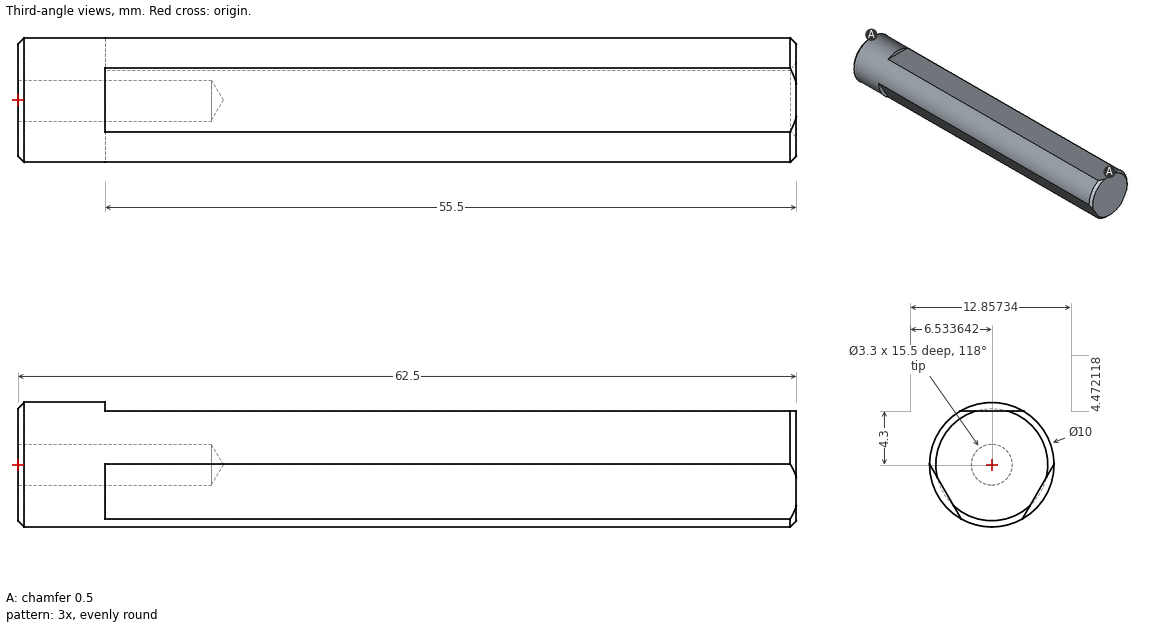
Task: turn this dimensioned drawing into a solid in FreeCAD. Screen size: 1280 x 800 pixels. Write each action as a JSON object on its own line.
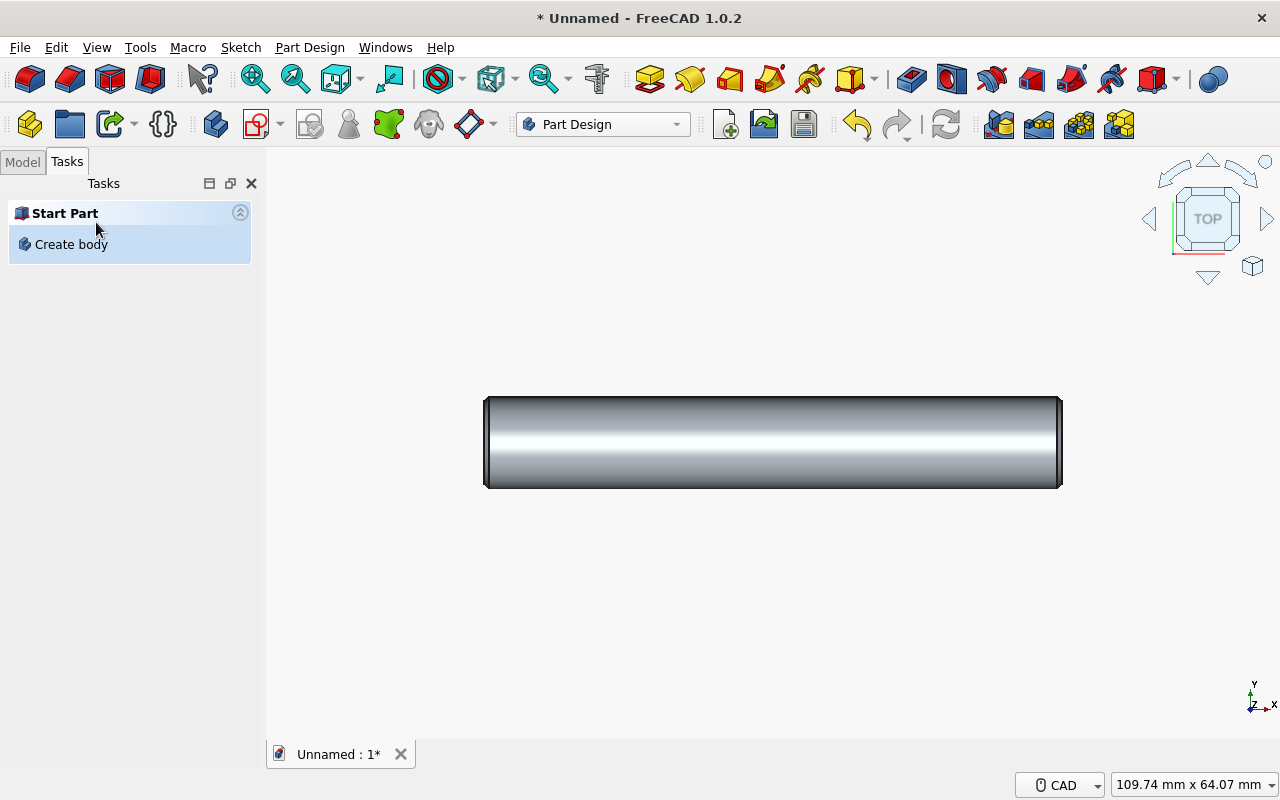
{"action": "key", "text": "0"}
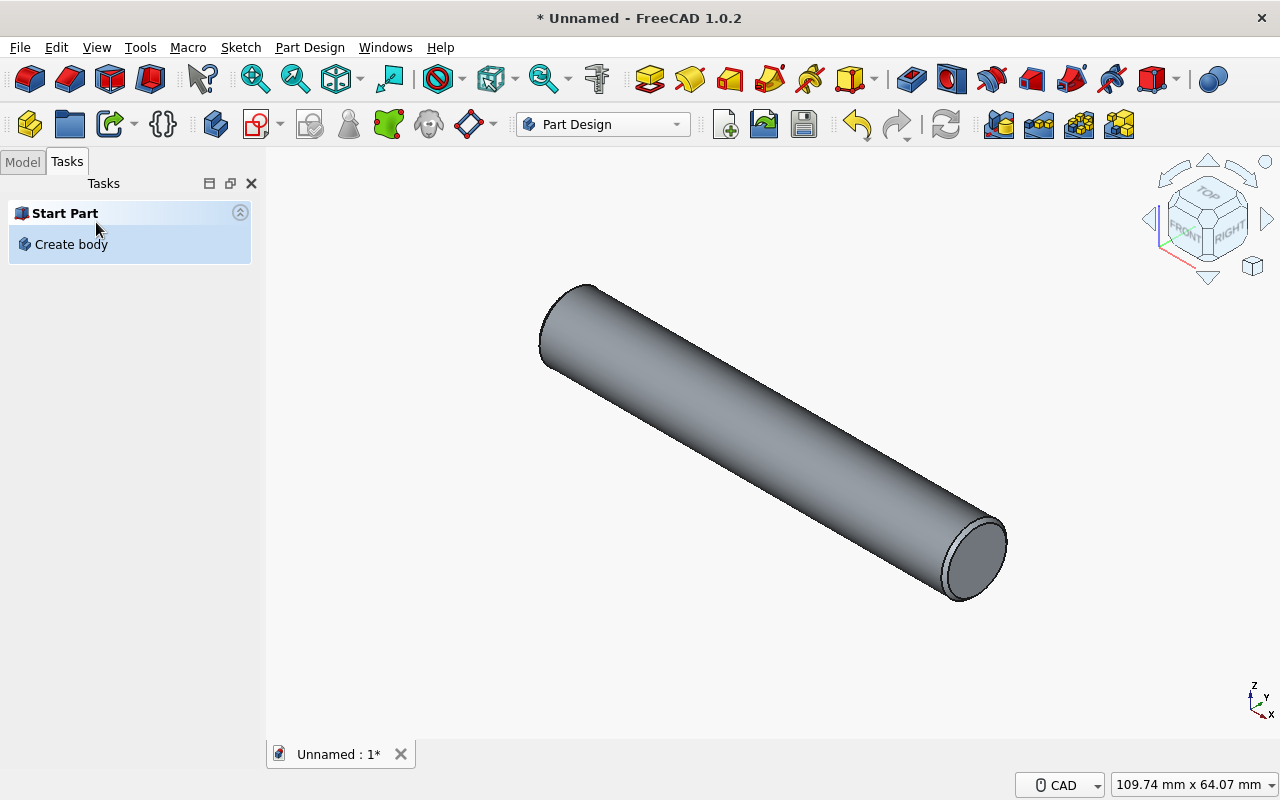
{"action": "left_click", "coordinate": [977, 560]}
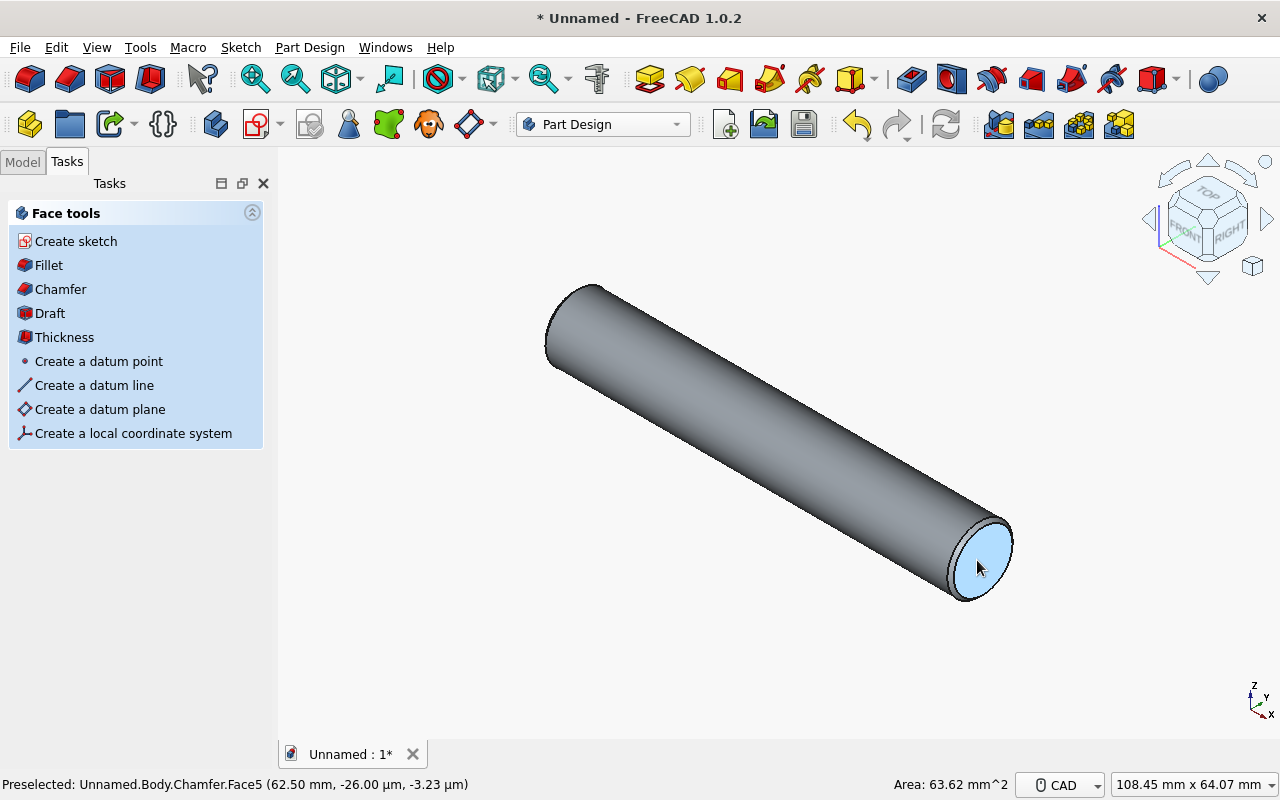
{"action": "left_click", "coordinate": [256, 124]}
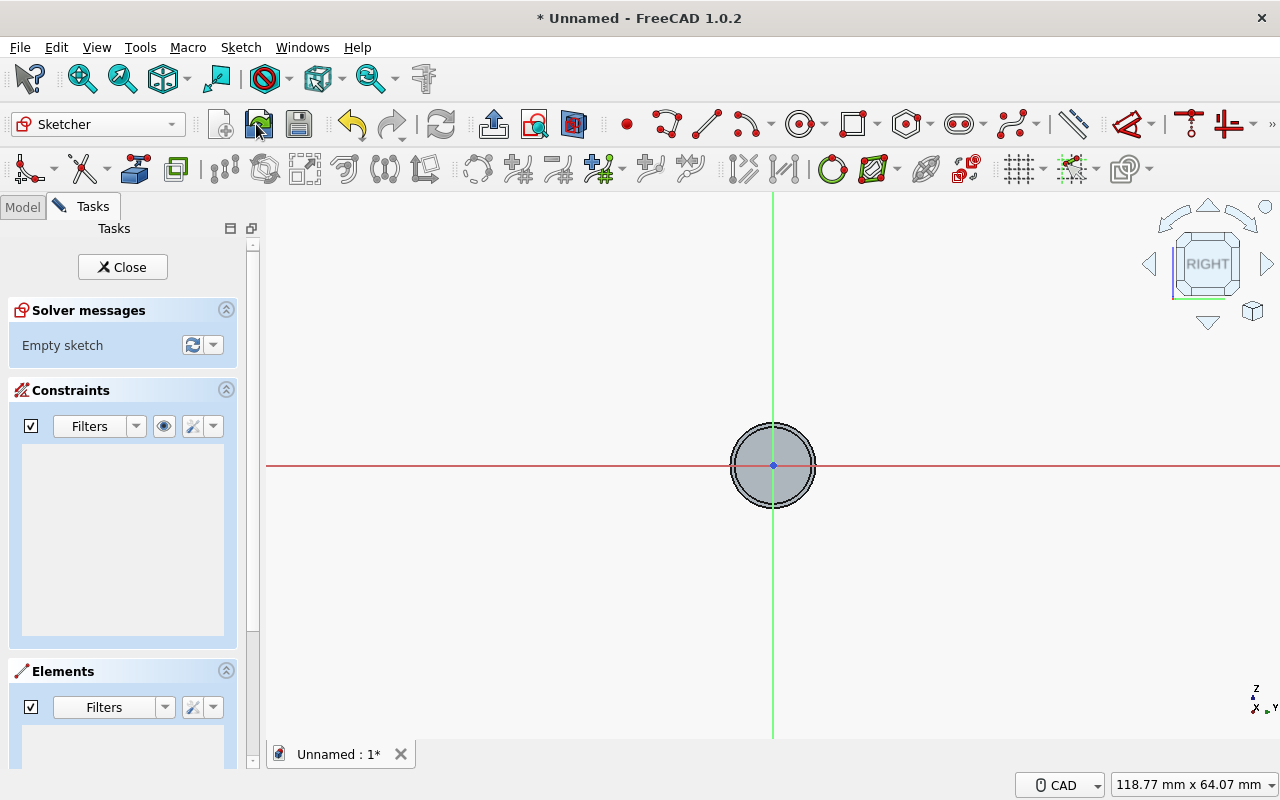
{"action": "scroll", "coordinate": [789, 419], "scroll_direction": "up", "scroll_amount": 8}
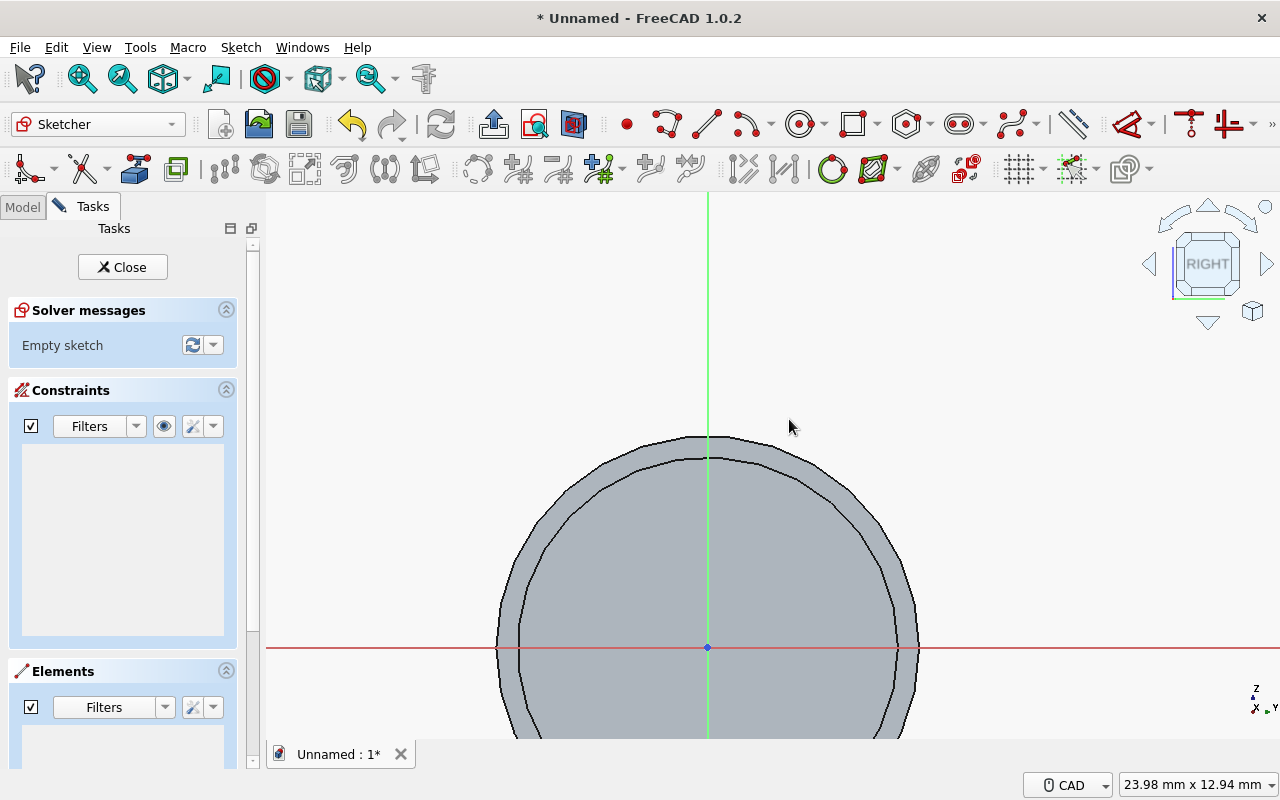
{"action": "left_click", "coordinate": [854, 124]}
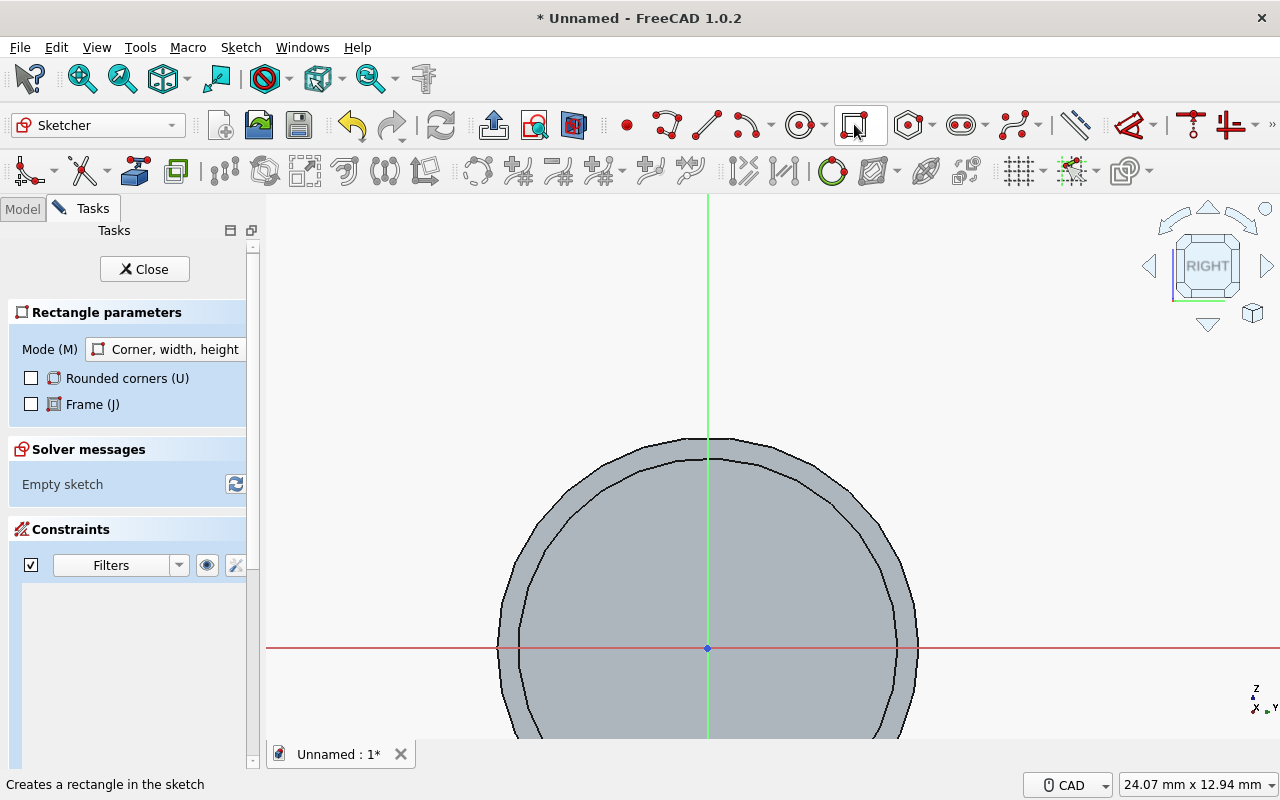
{"action": "left_click", "coordinate": [433, 278]}
{"action": "mouse_move", "coordinate": [974, 467]}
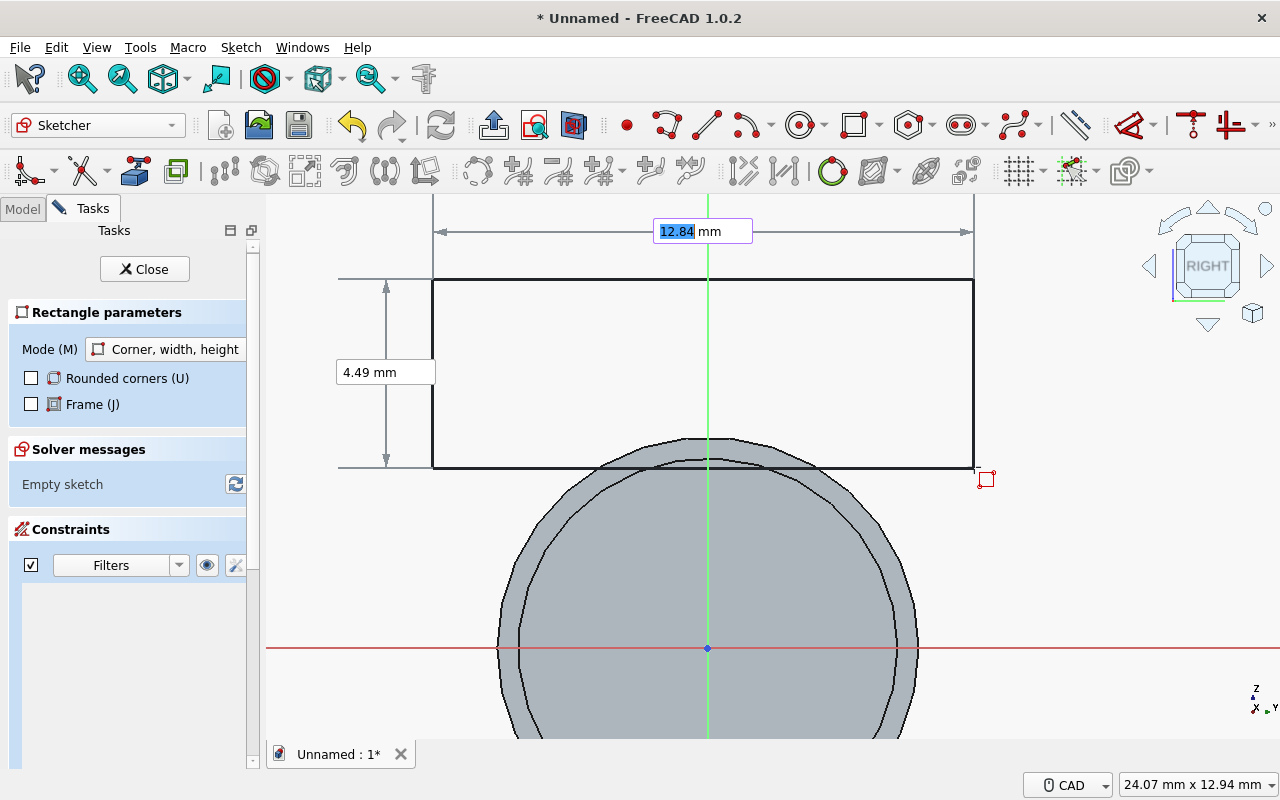
{"action": "type", "text": "12.85734"}
{"action": "key", "text": "Tab"}
{"action": "type", "text": "4.472118"}
{"action": "key", "text": "Return"}
{"action": "key", "text": "Escape"}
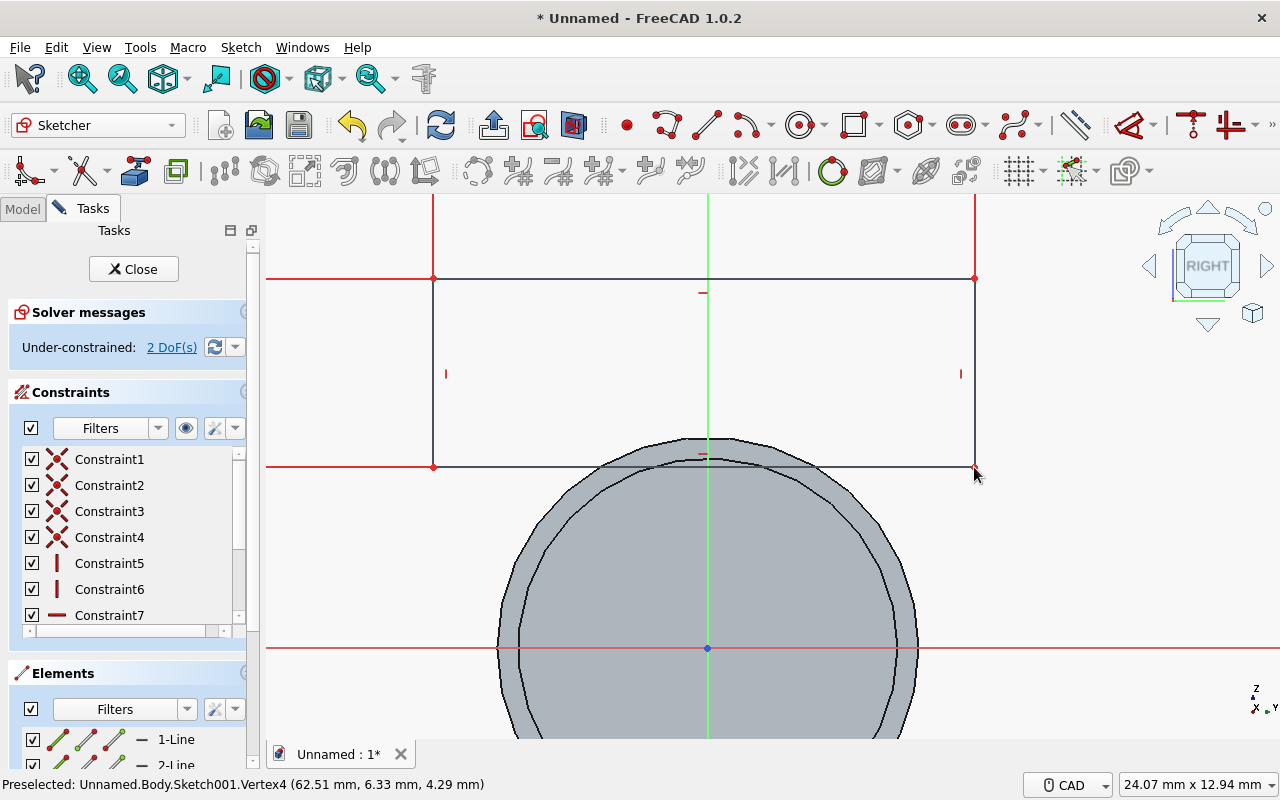
{"action": "left_click", "coordinate": [1130, 126]}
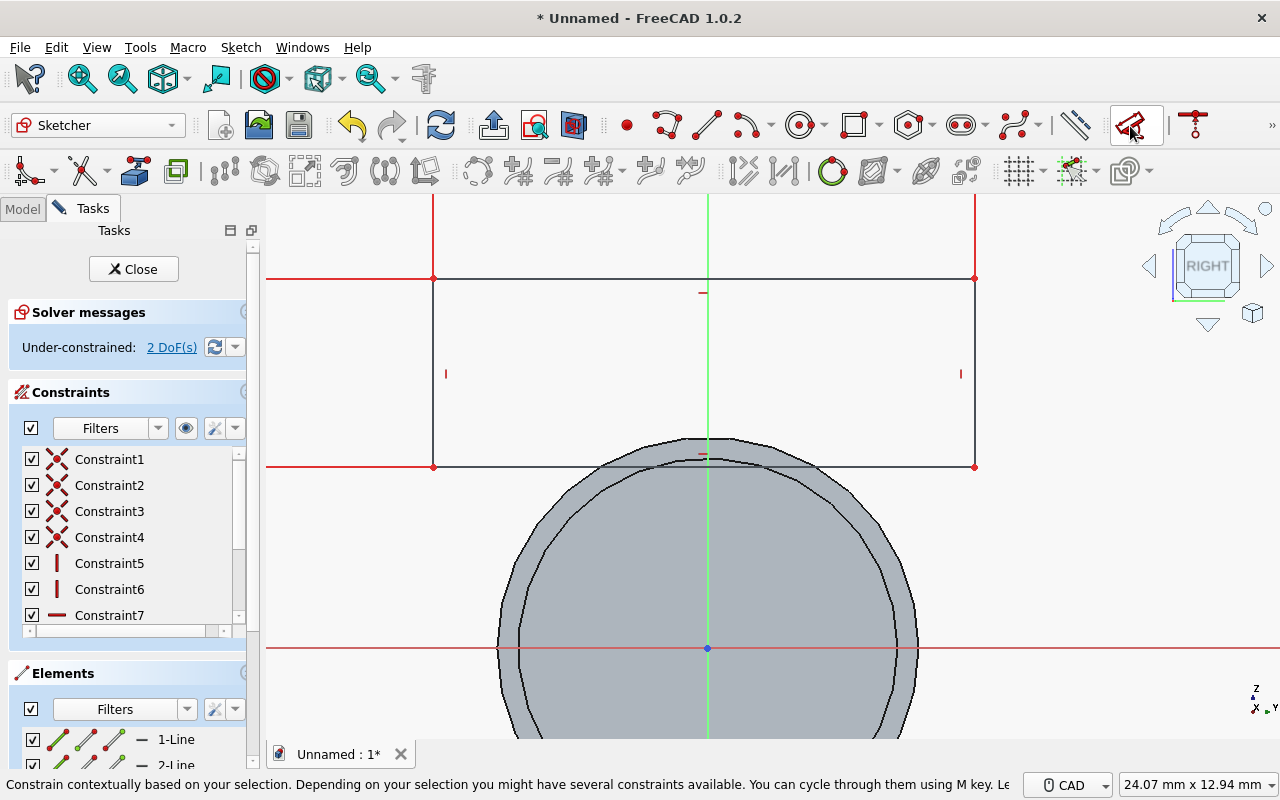
{"action": "left_click", "coordinate": [433, 467]}
{"action": "left_click", "coordinate": [399, 558]}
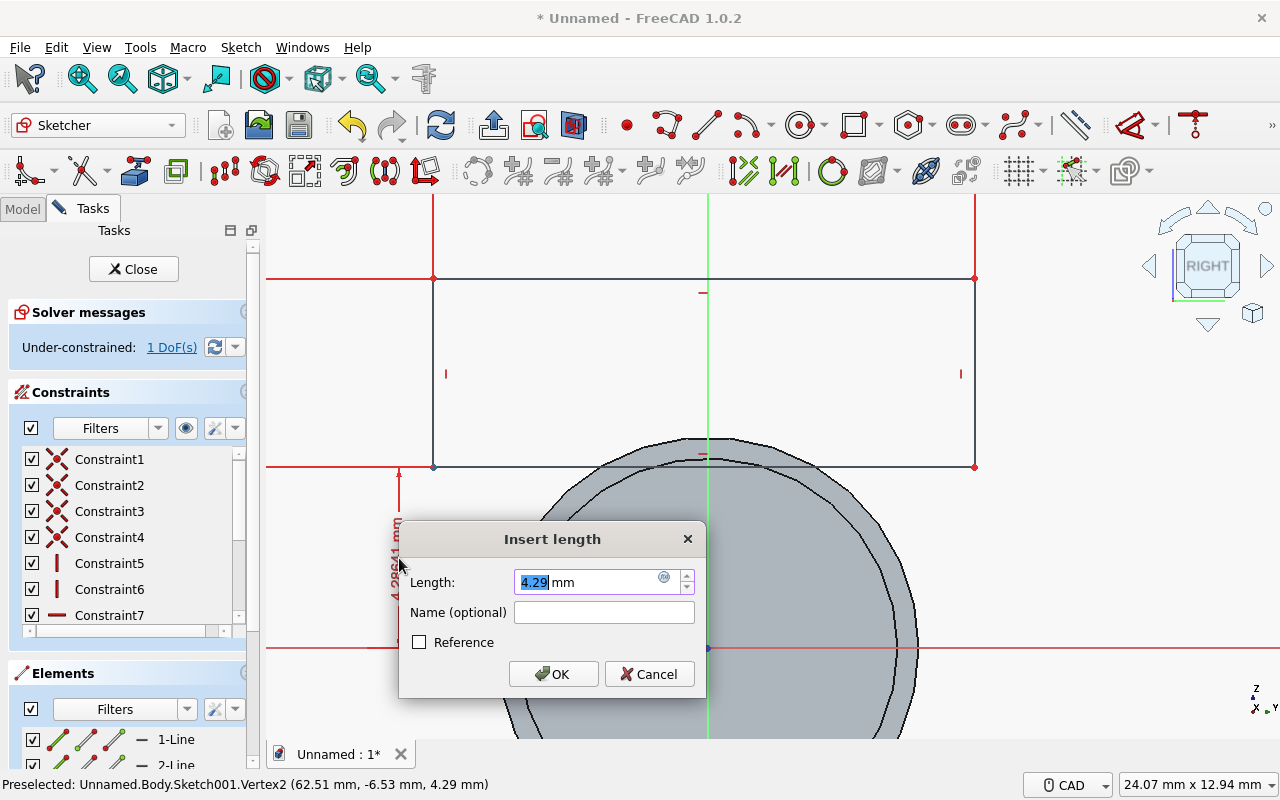
{"action": "type", "text": "4.3"}
{"action": "key", "text": "Return"}